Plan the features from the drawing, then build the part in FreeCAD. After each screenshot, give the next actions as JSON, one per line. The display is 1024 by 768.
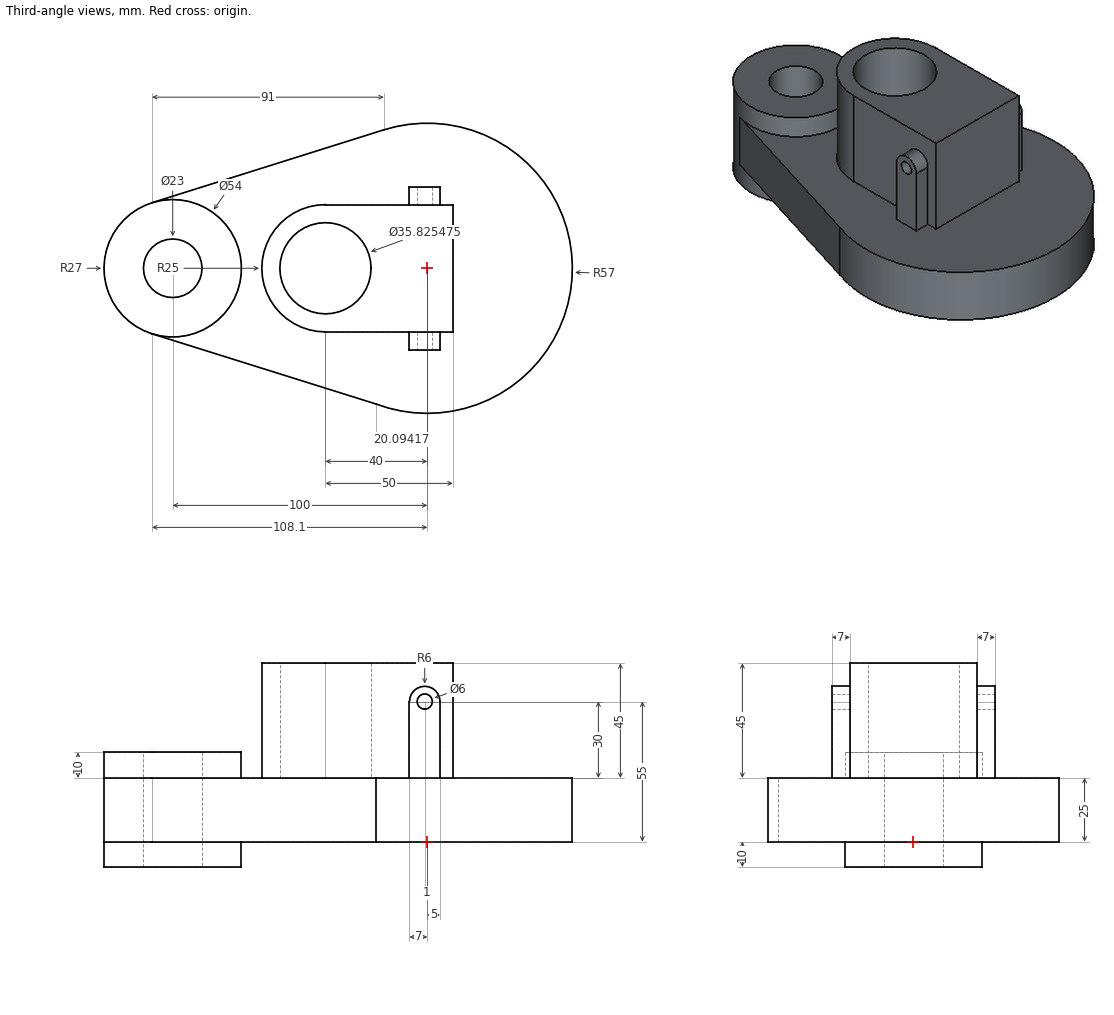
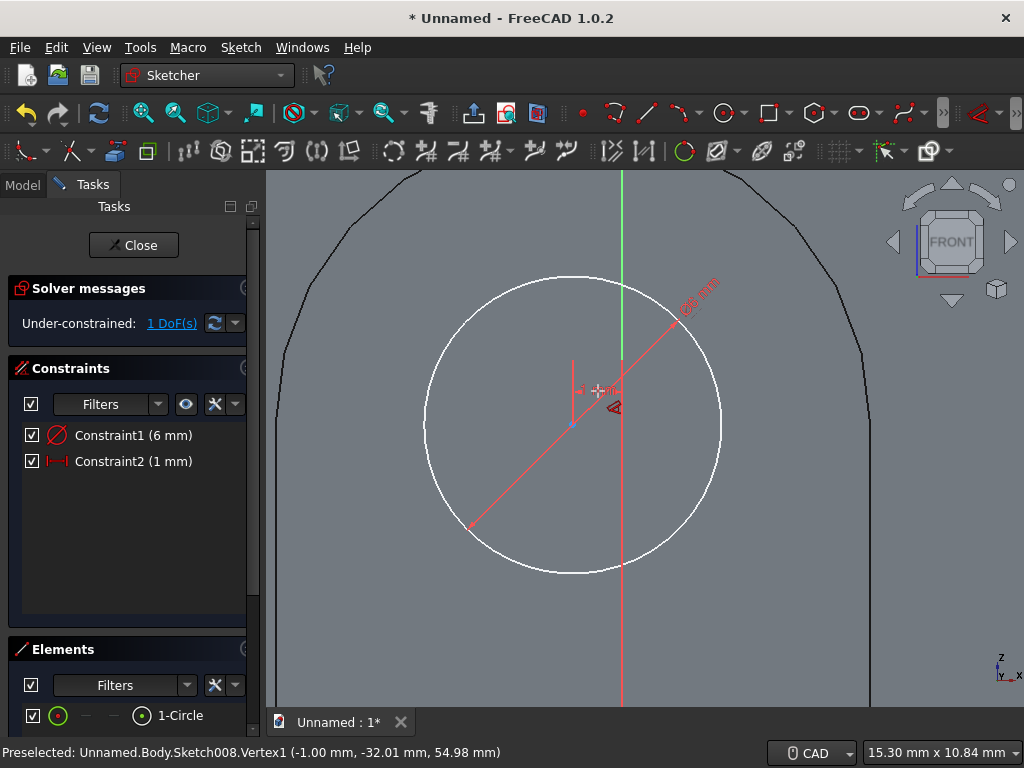
{"action": "left_click", "coordinate": [573, 425]}
{"action": "left_click", "coordinate": [656, 494]}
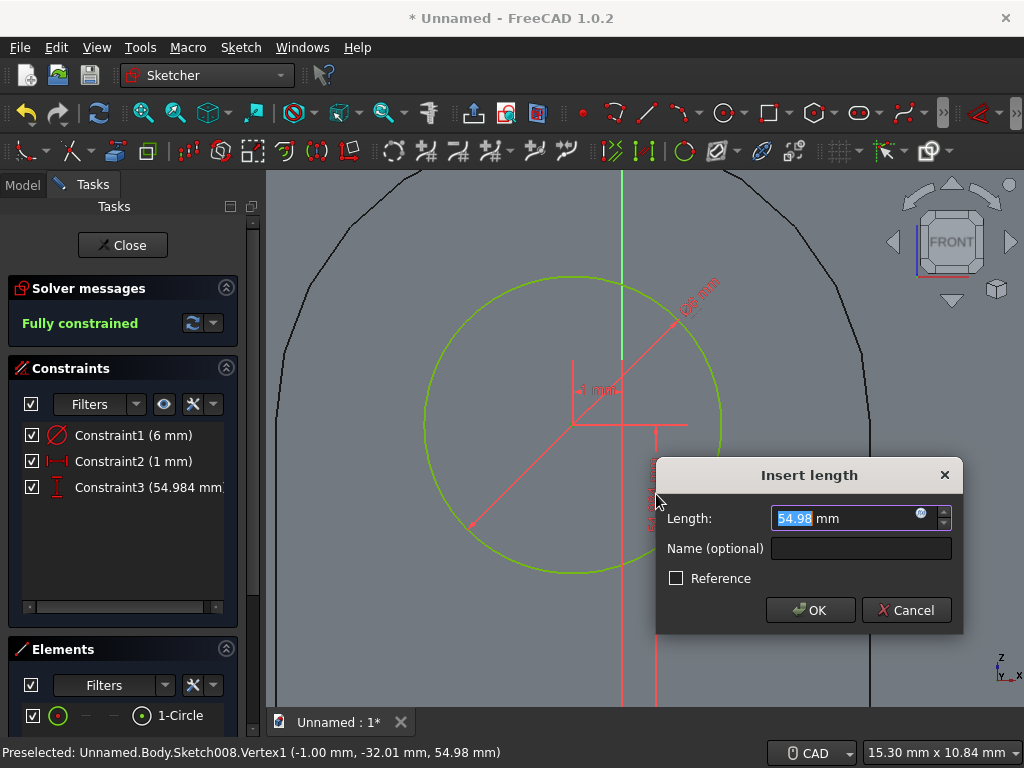
{"action": "type", "text": "55"}
{"action": "key", "text": "Return"}
{"action": "key", "text": "Escape"}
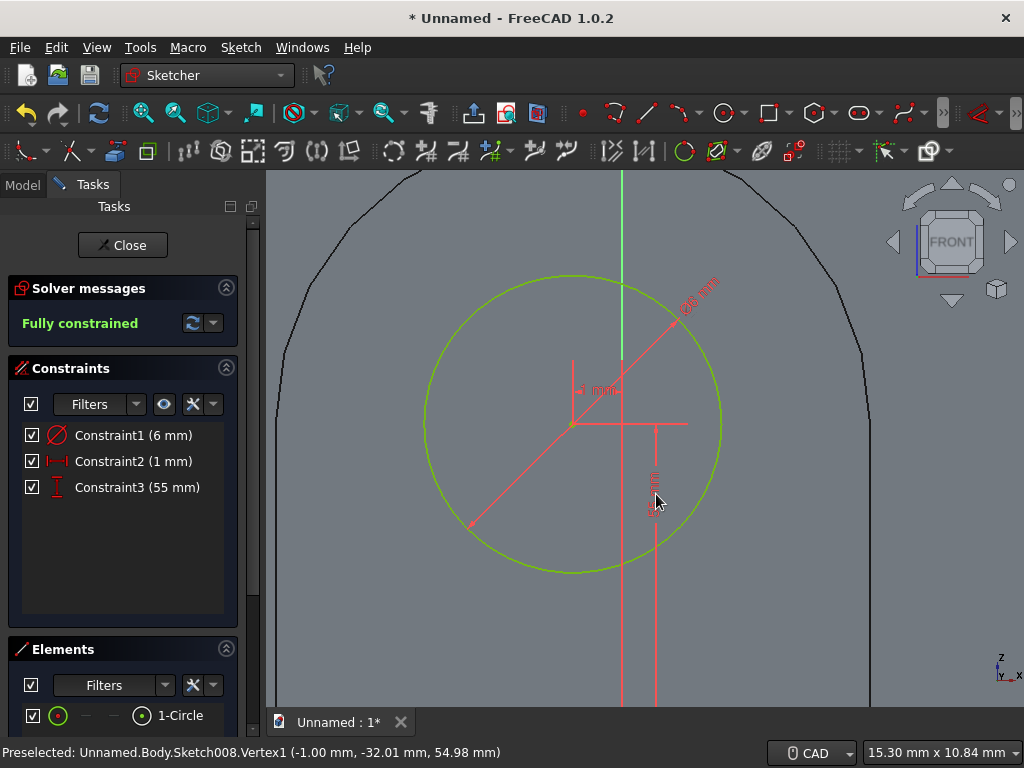
{"action": "left_click", "coordinate": [123, 245]}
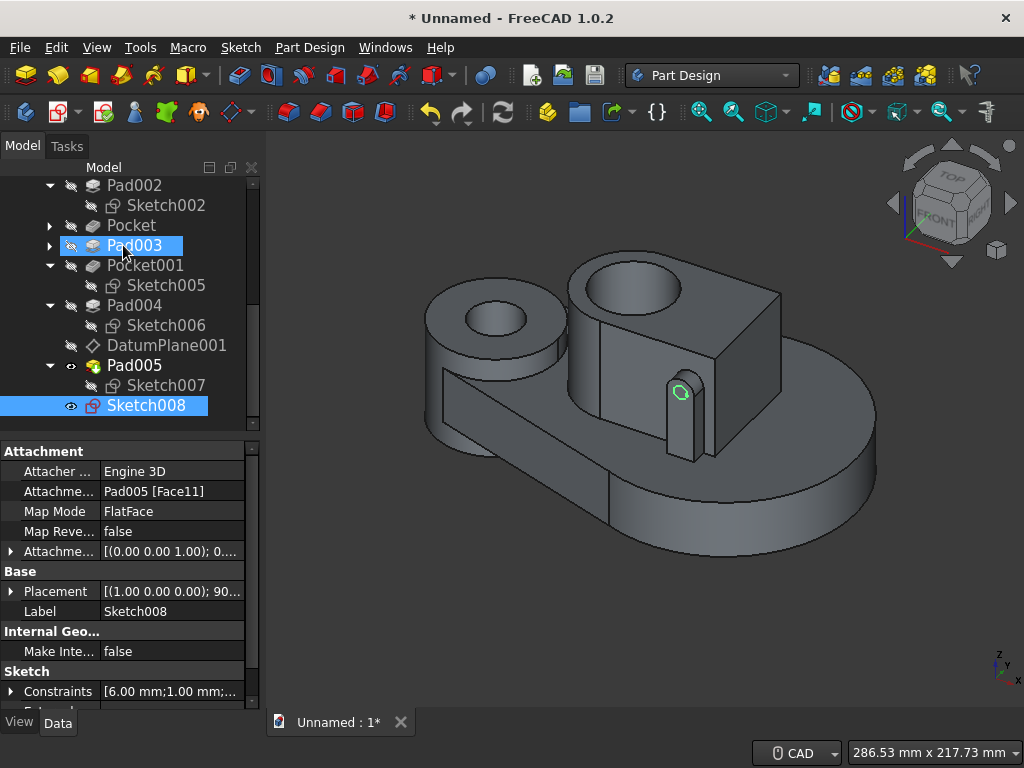
{"action": "left_click", "coordinate": [240, 76]}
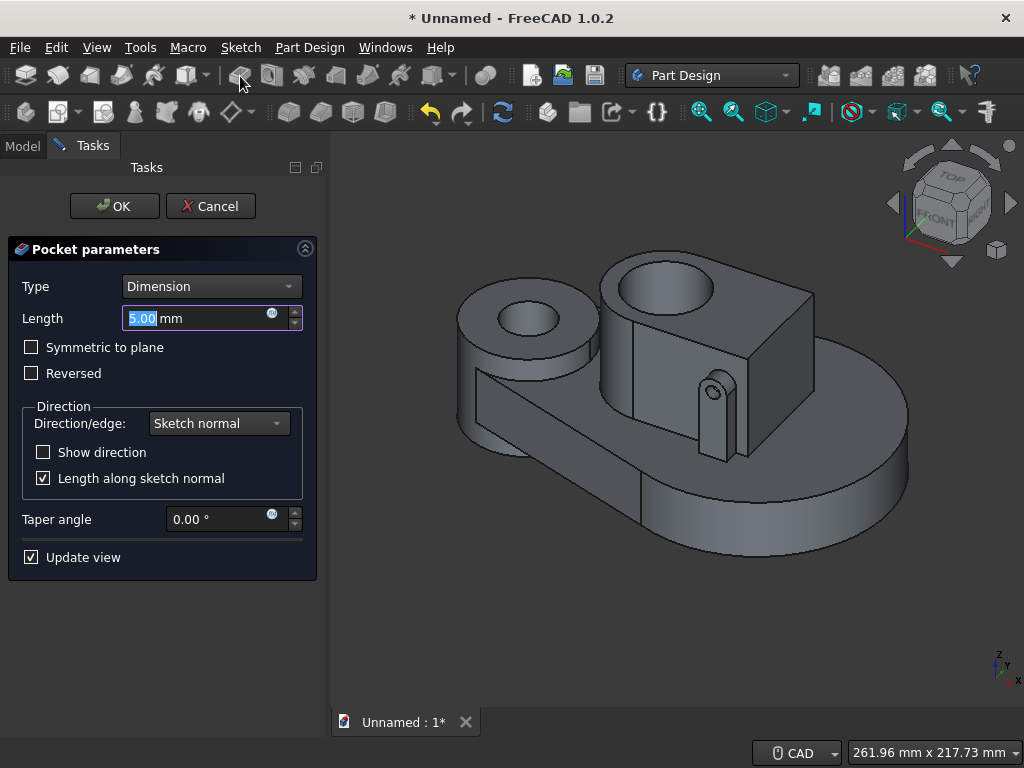
{"action": "type", "text": "7"}
{"action": "key", "text": "Tab"}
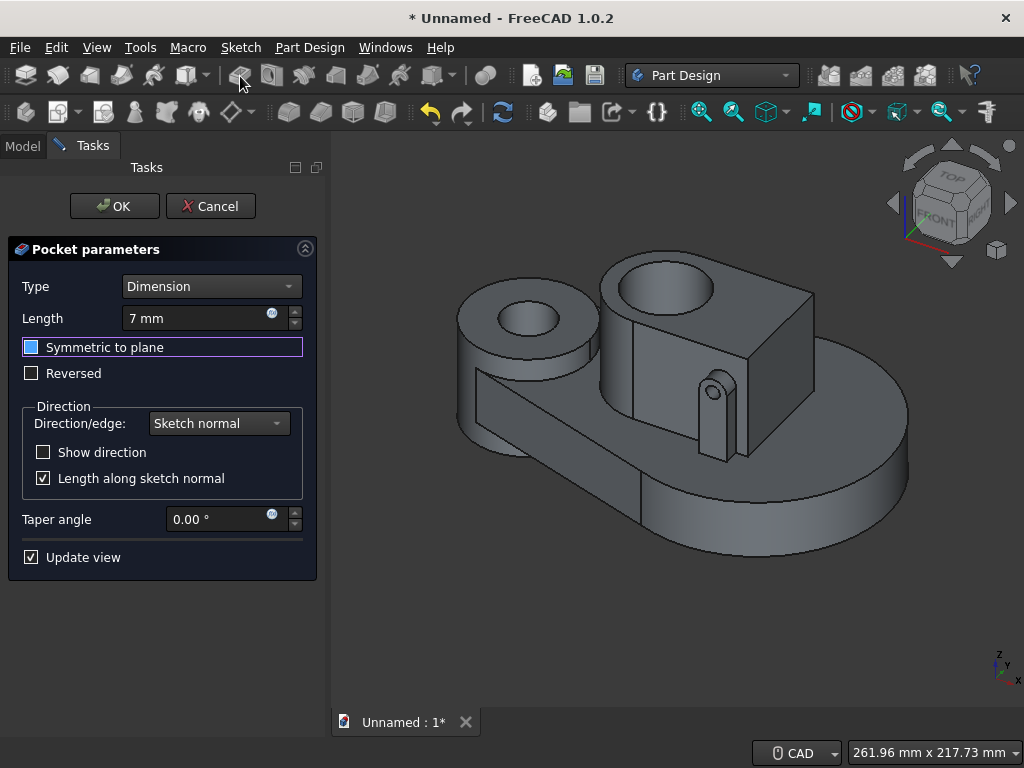
{"action": "left_click", "coordinate": [115, 206]}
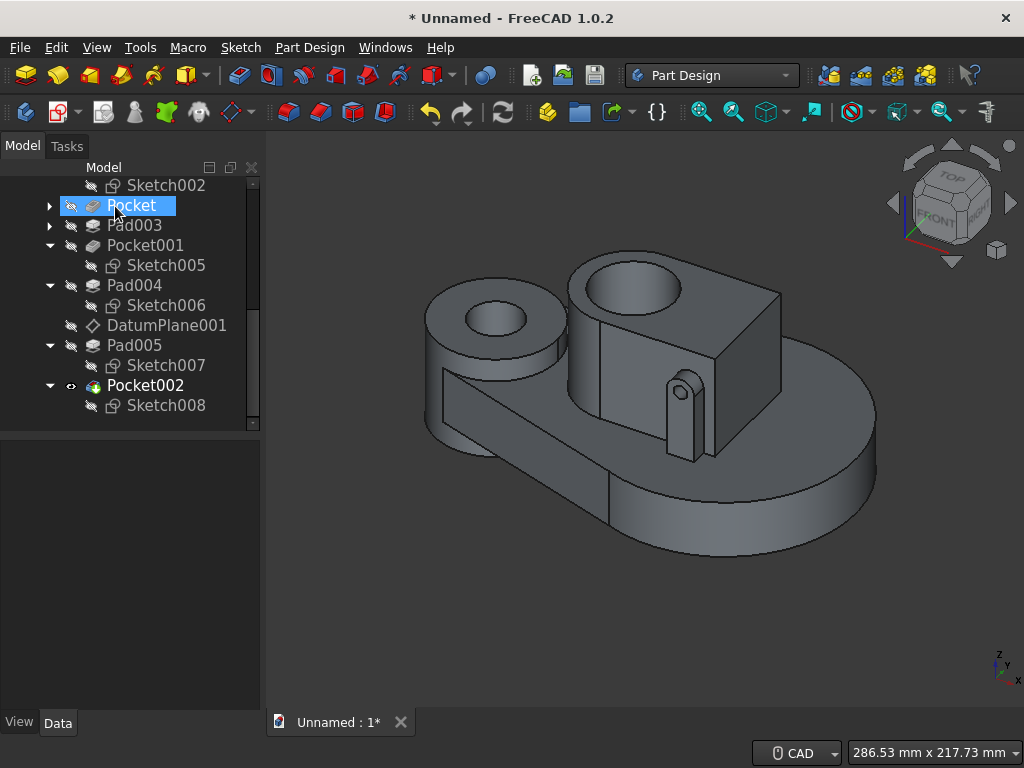
{"action": "key", "text": "4"}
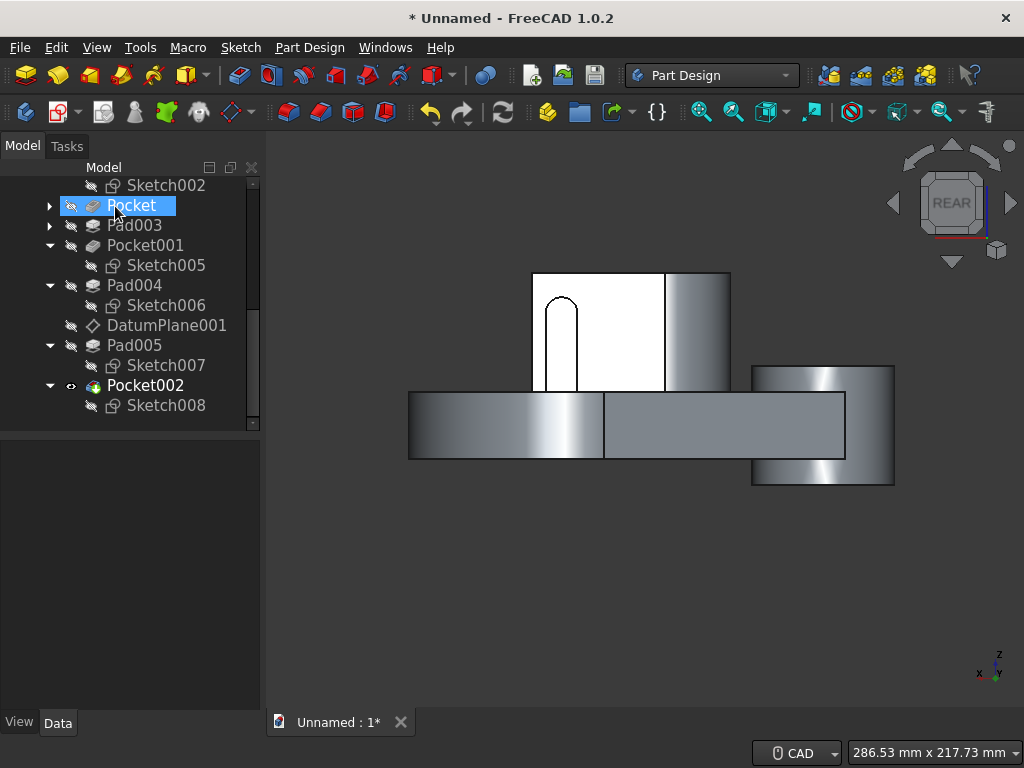
{"action": "left_click", "coordinate": [618, 315]}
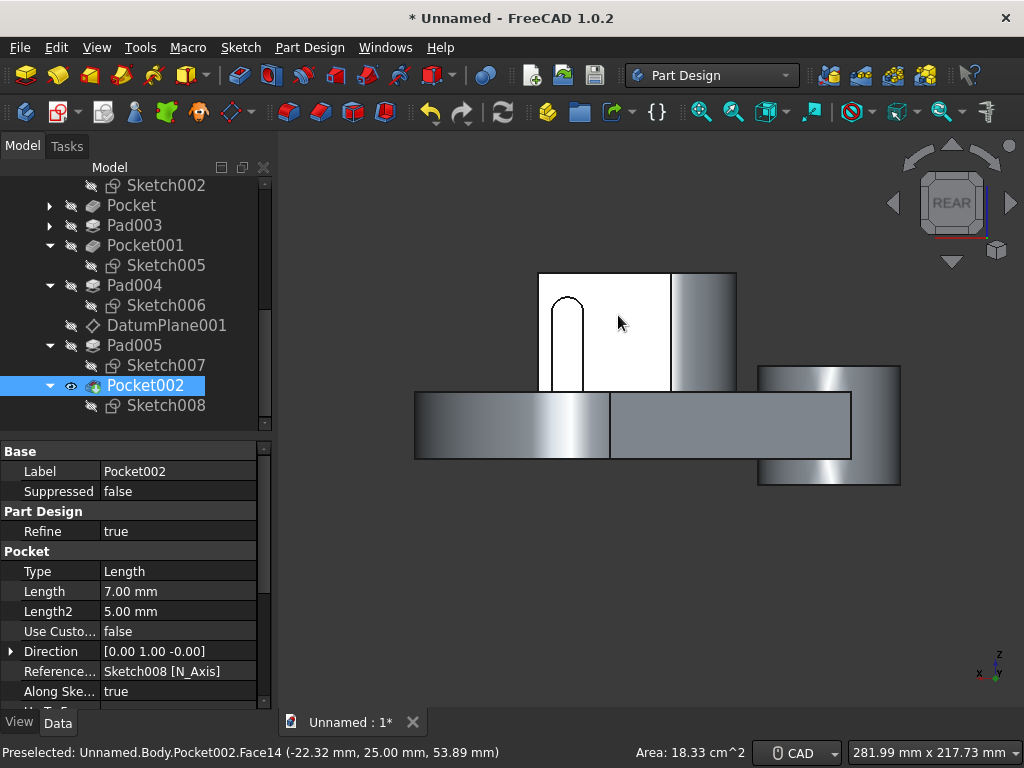
{"action": "left_click", "coordinate": [58, 112]}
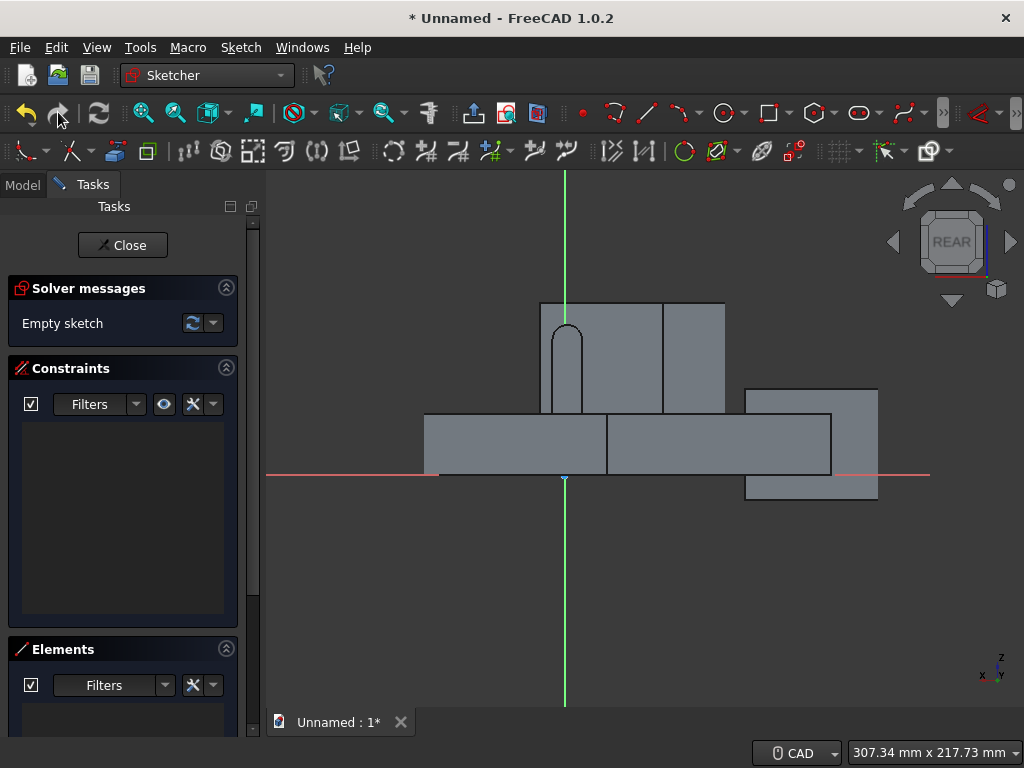
{"action": "scroll", "coordinate": [567, 335], "scroll_direction": "up", "scroll_amount": 15}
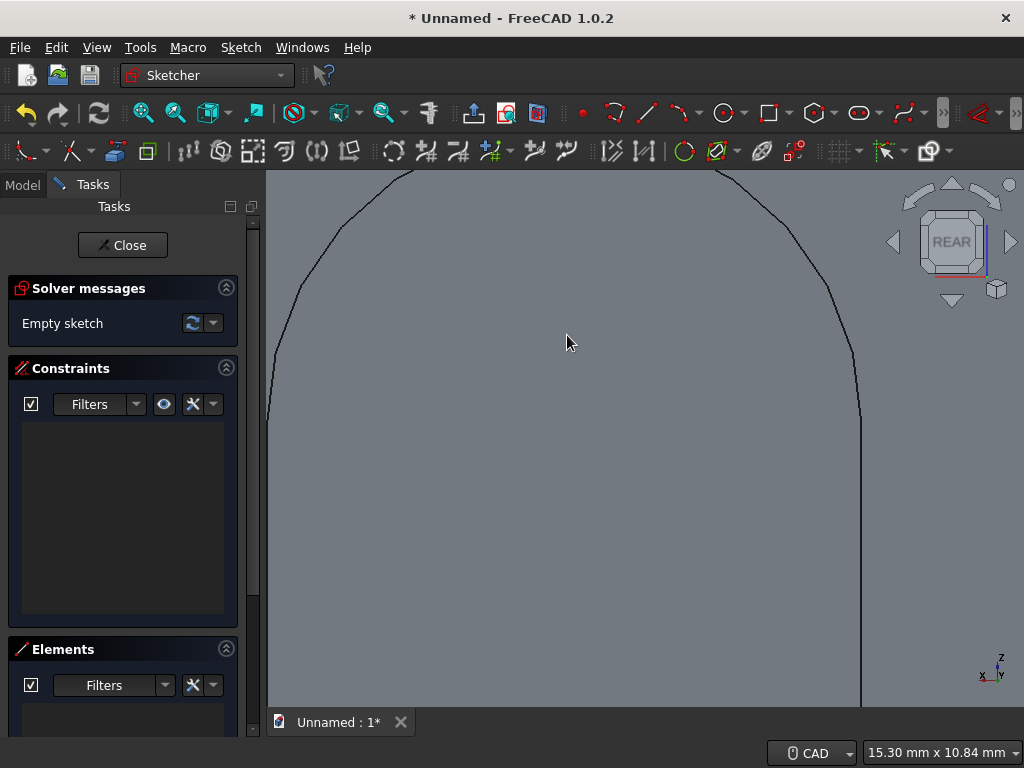
{"action": "key", "text": "g c"}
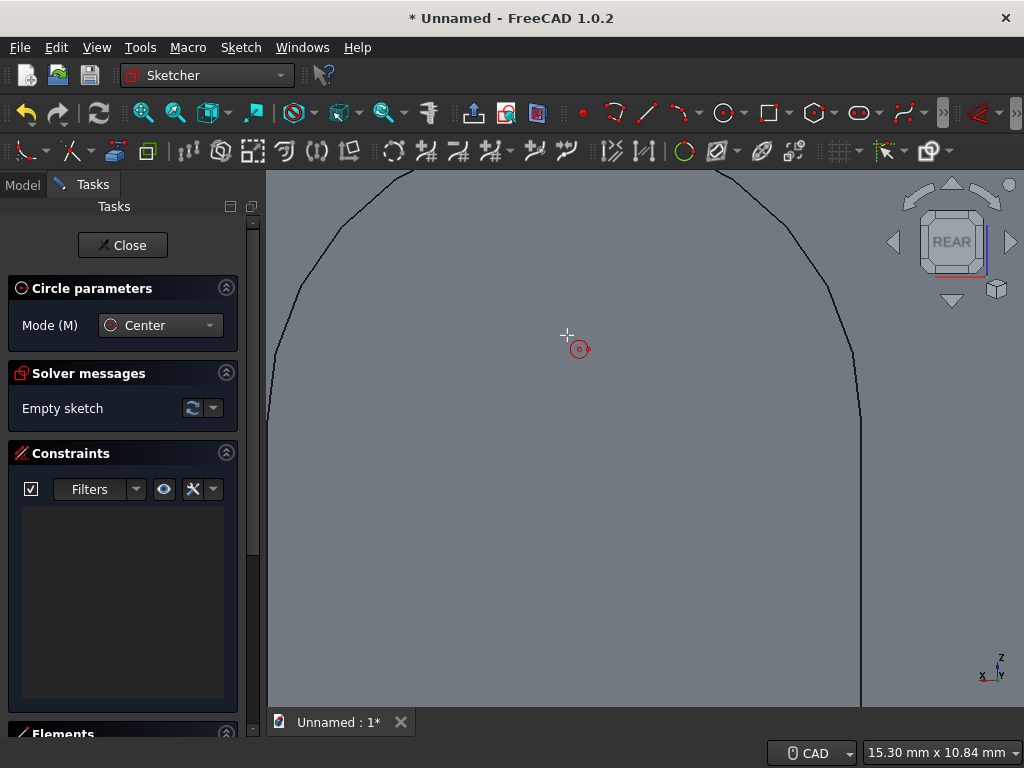
{"action": "left_click", "coordinate": [564, 424]}
{"action": "left_click", "coordinate": [669, 319]}
{"action": "key", "text": "Escape"}